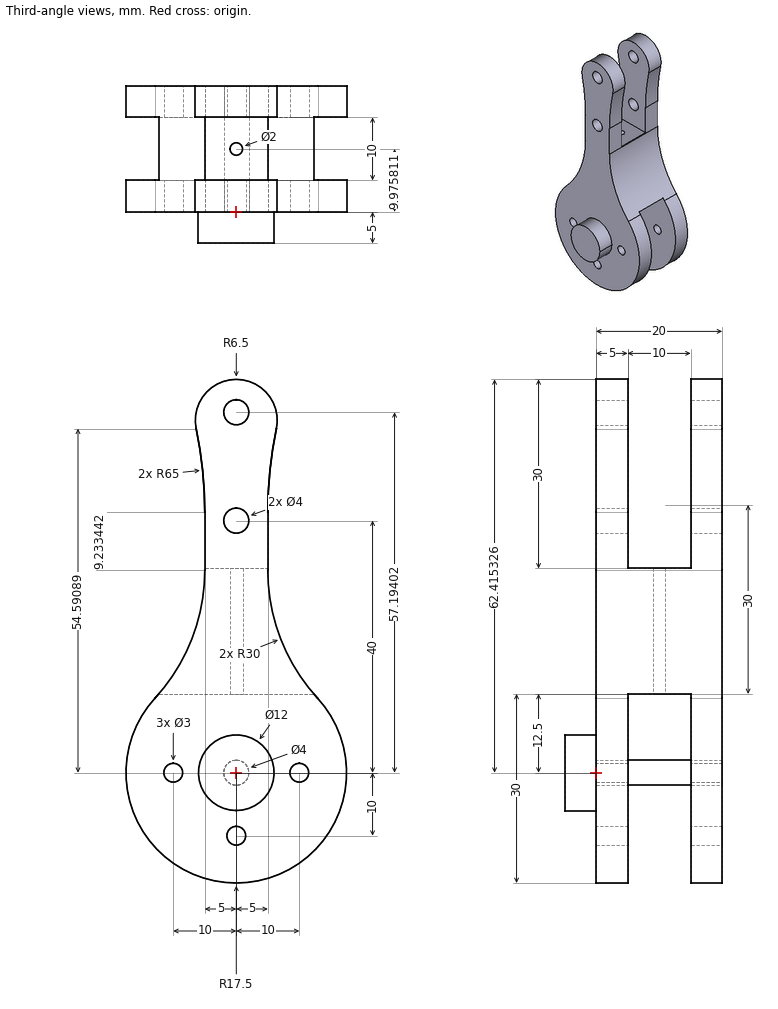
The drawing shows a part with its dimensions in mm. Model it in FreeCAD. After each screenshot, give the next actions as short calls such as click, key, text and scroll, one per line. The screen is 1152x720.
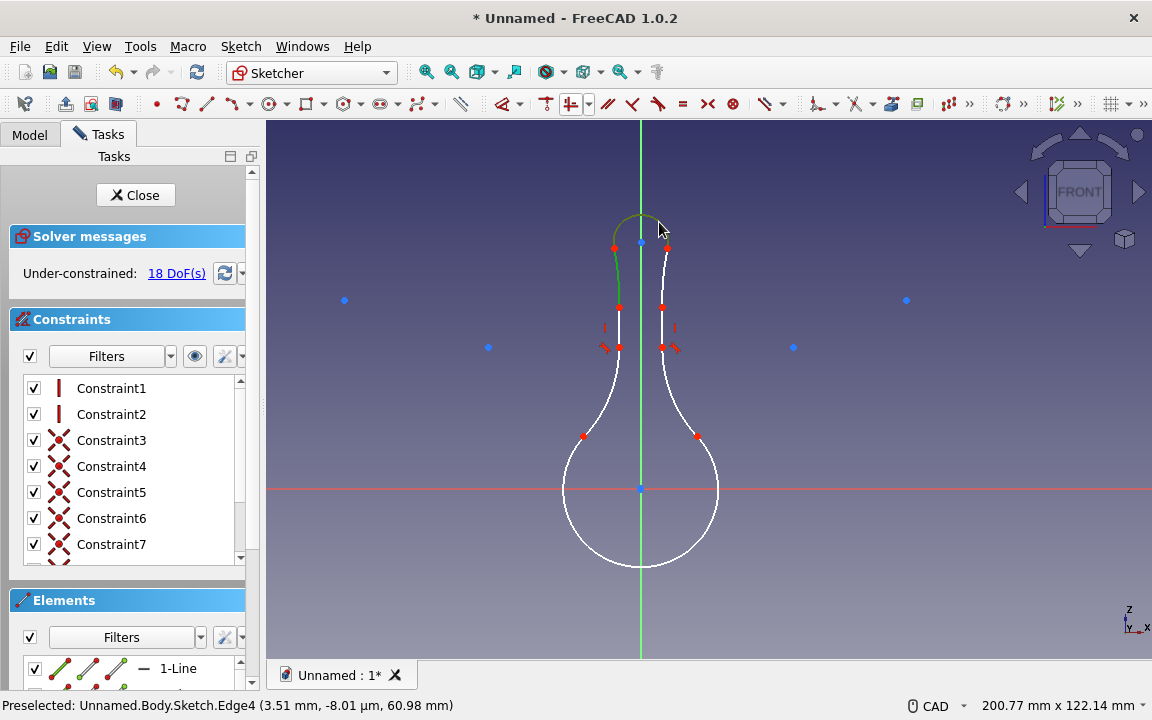
click(658, 104)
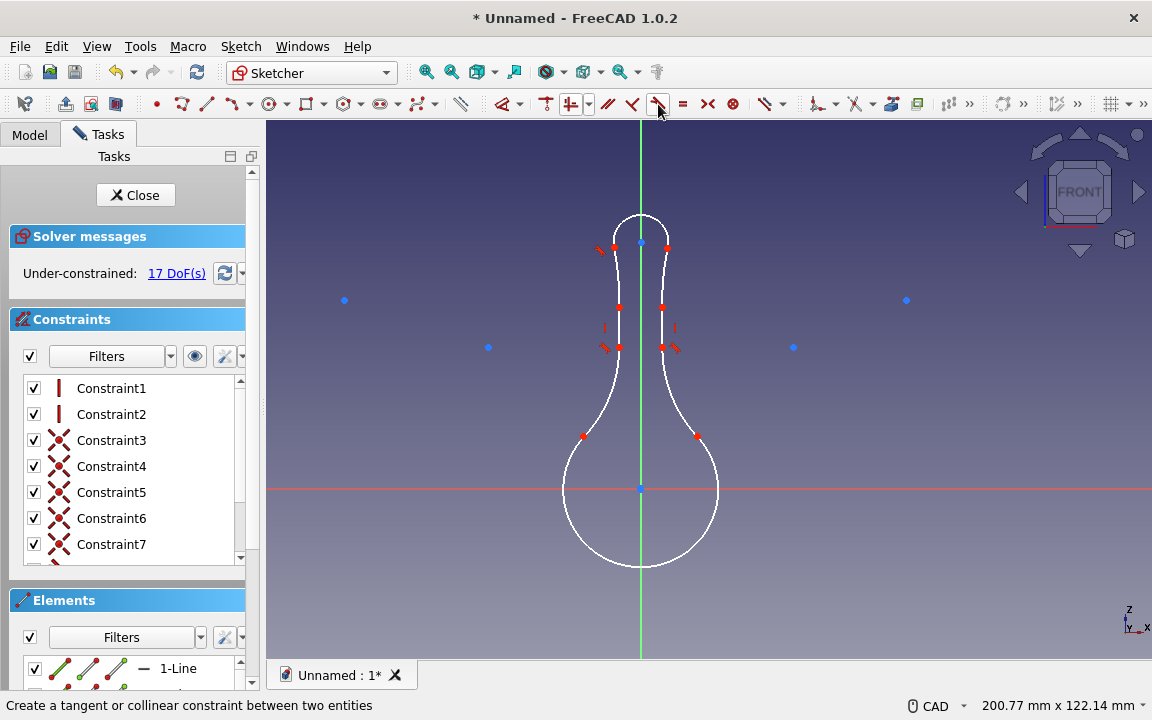
click(660, 222)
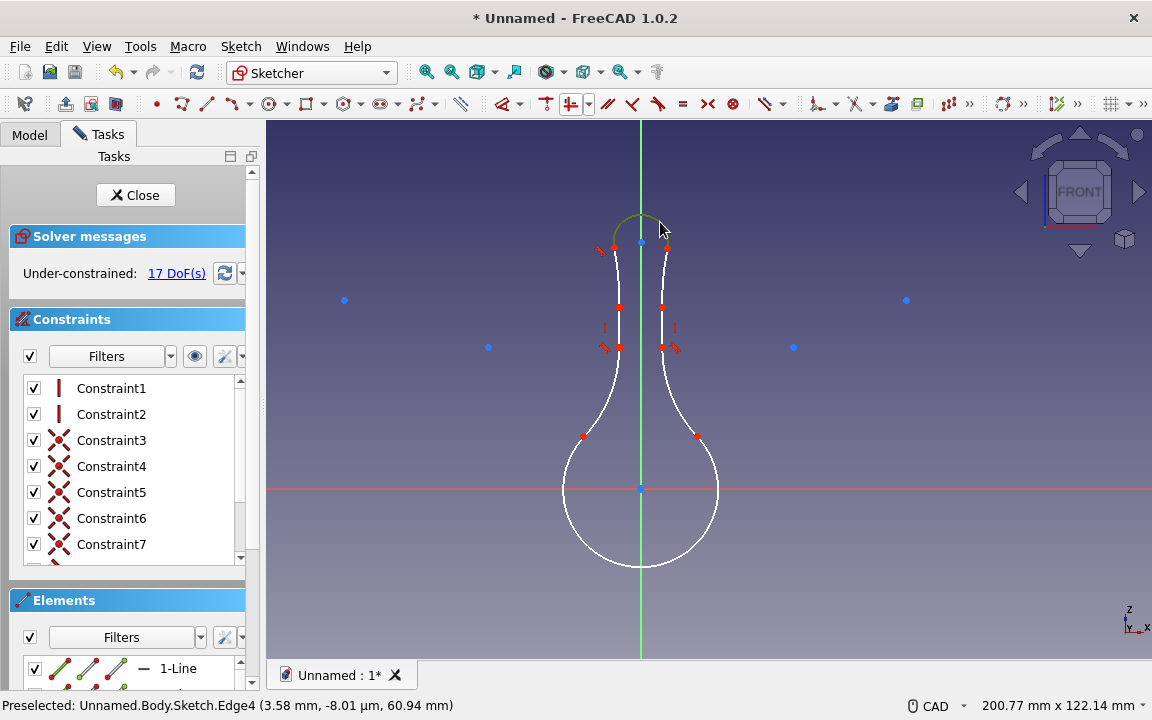
click(665, 266)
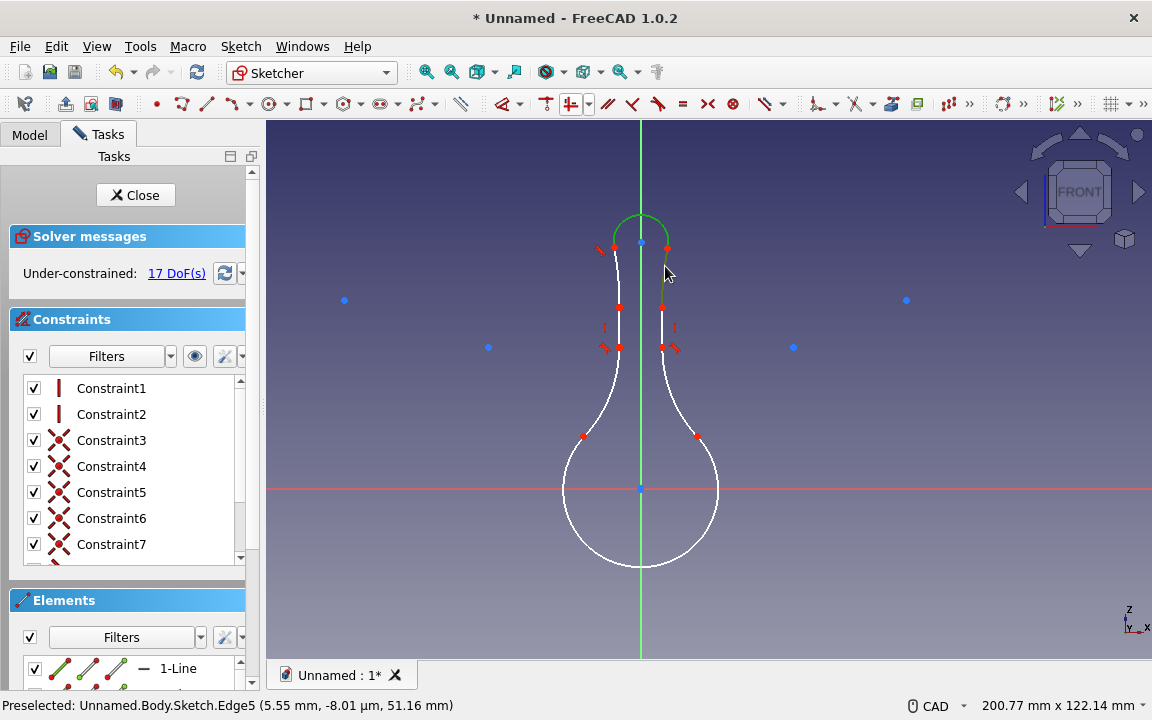
click(658, 104)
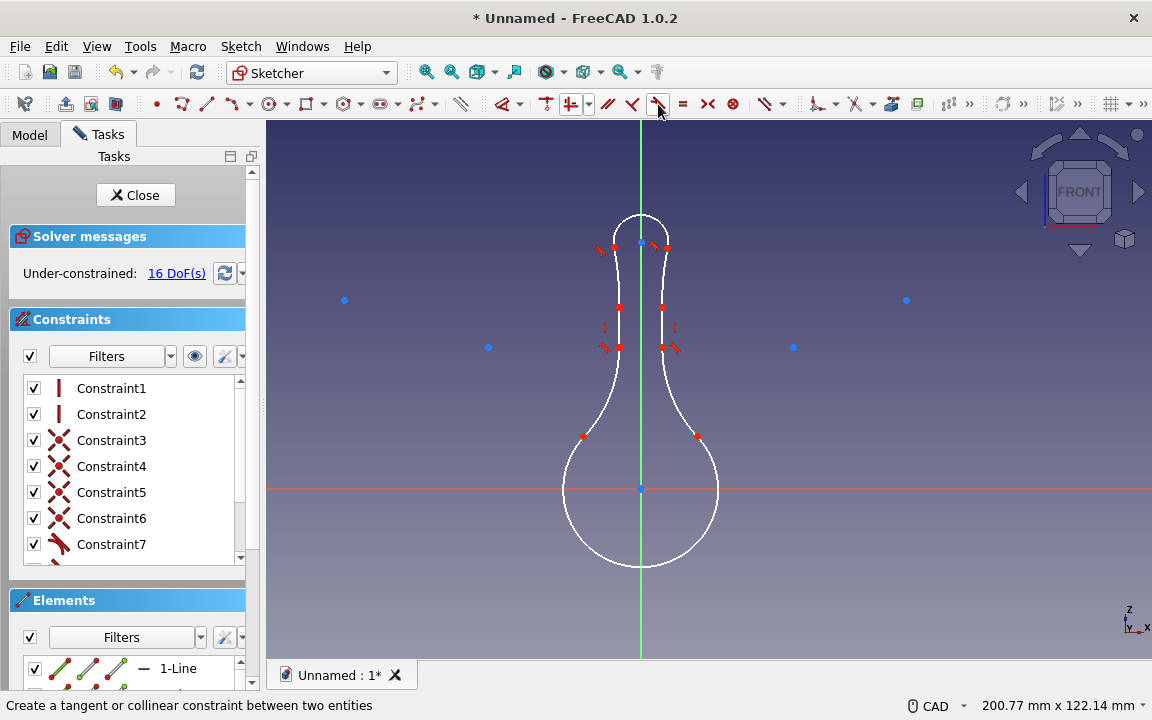
click(666, 377)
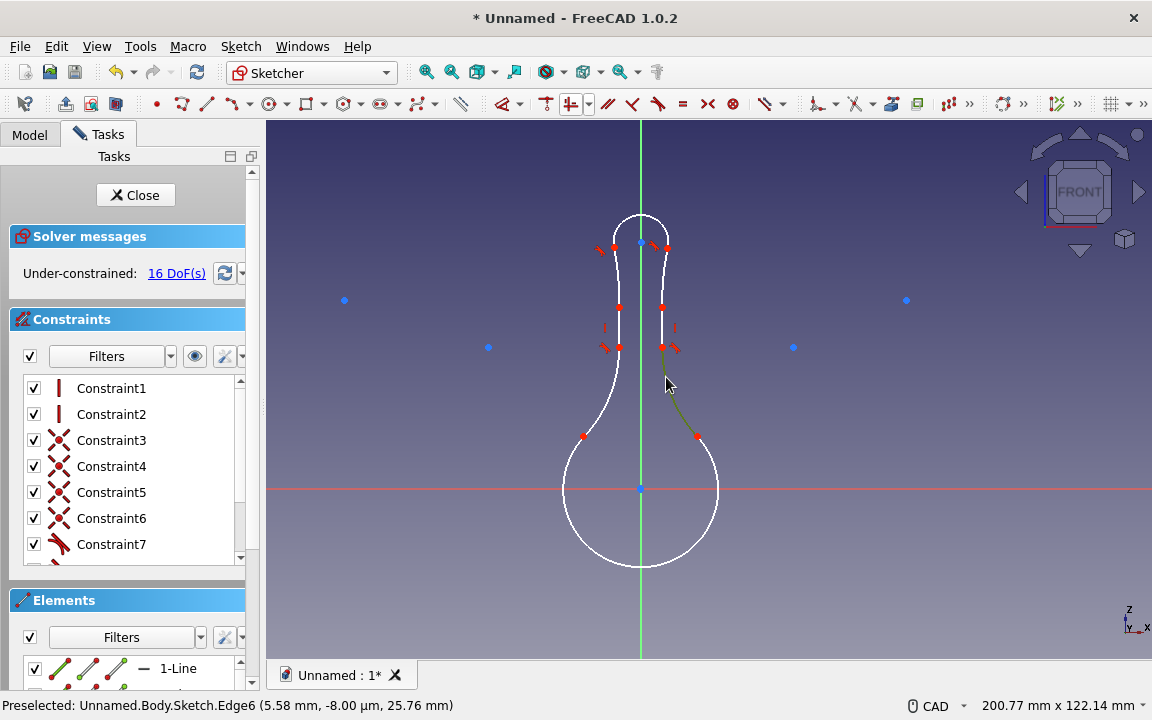
click(579, 536)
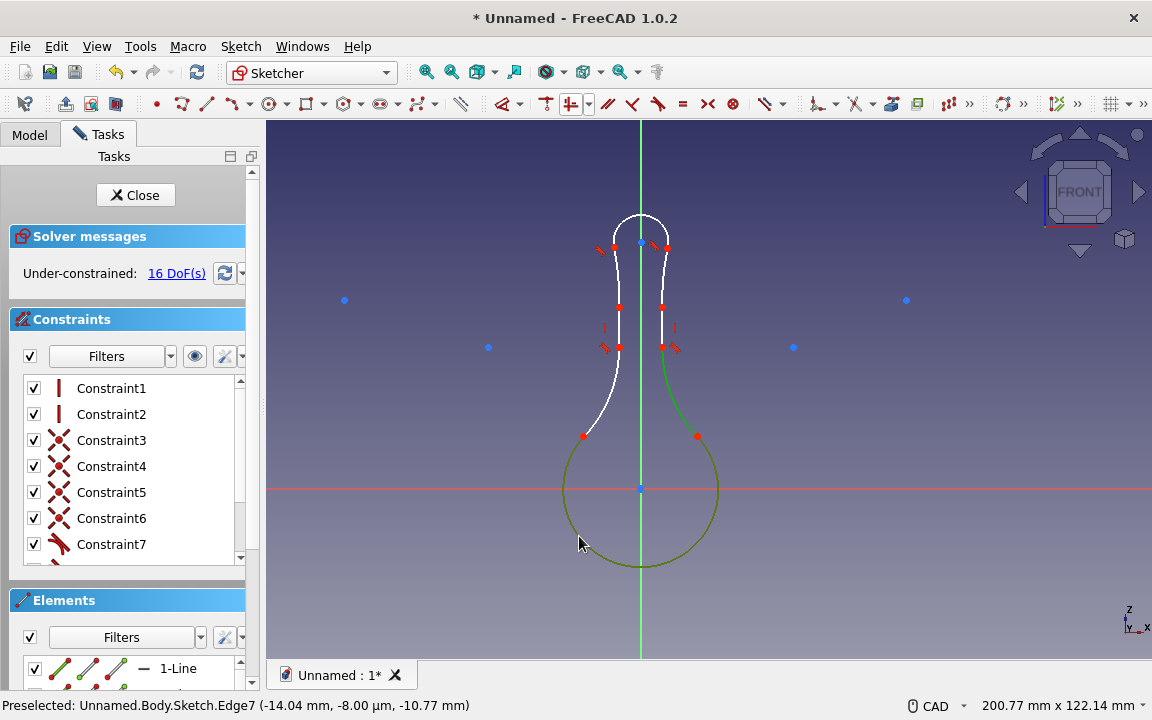
click(658, 104)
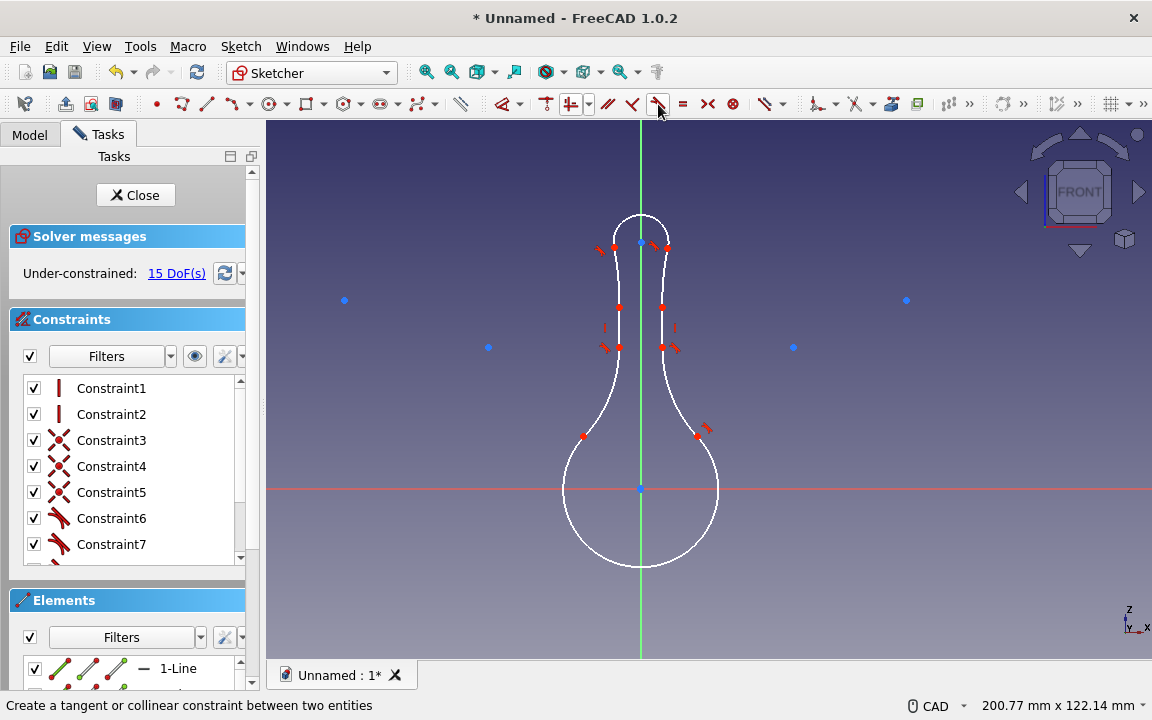
click(579, 536)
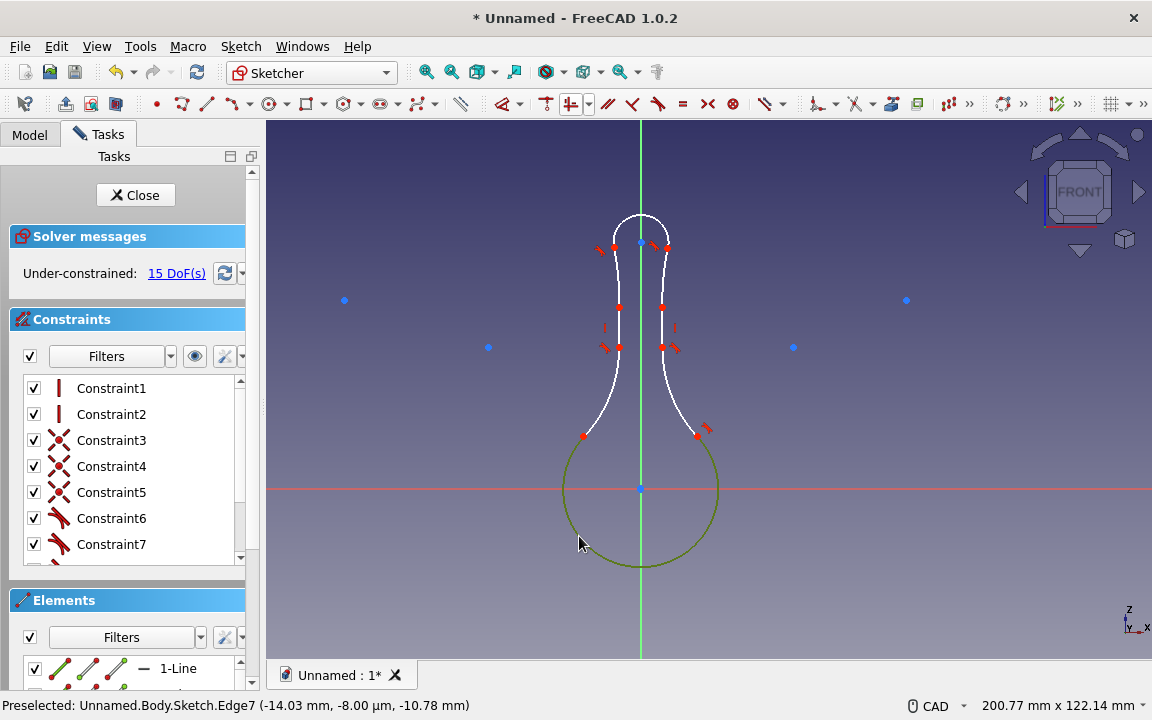
click(601, 413)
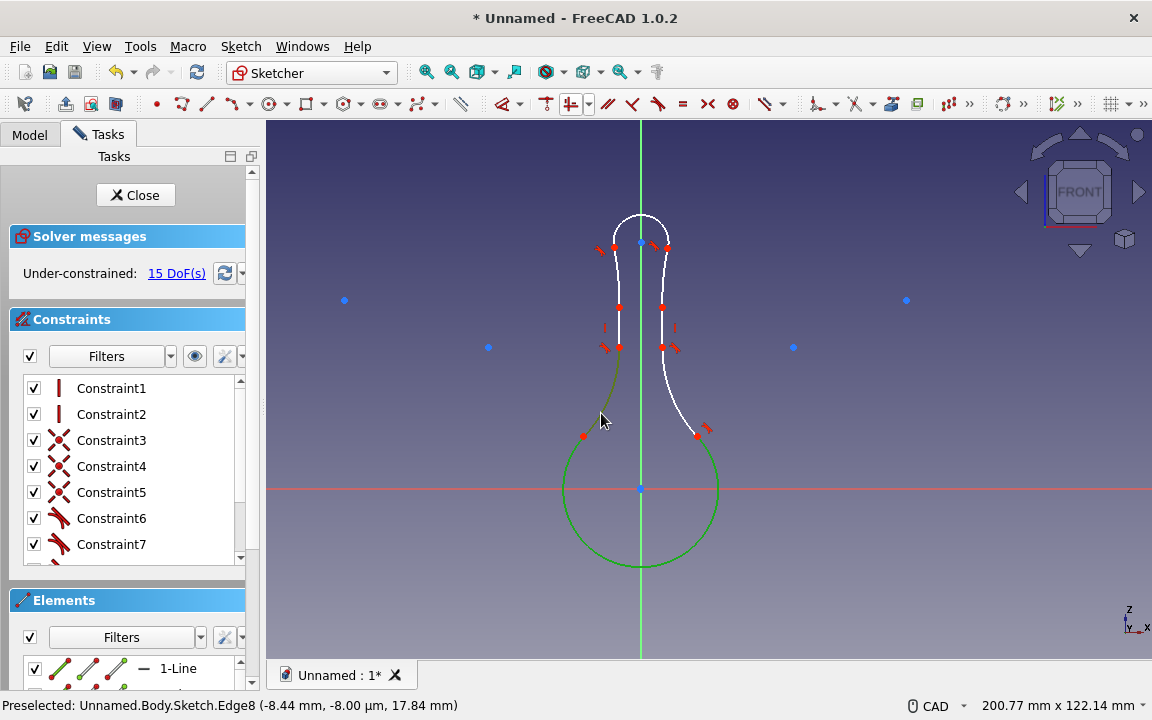
click(658, 104)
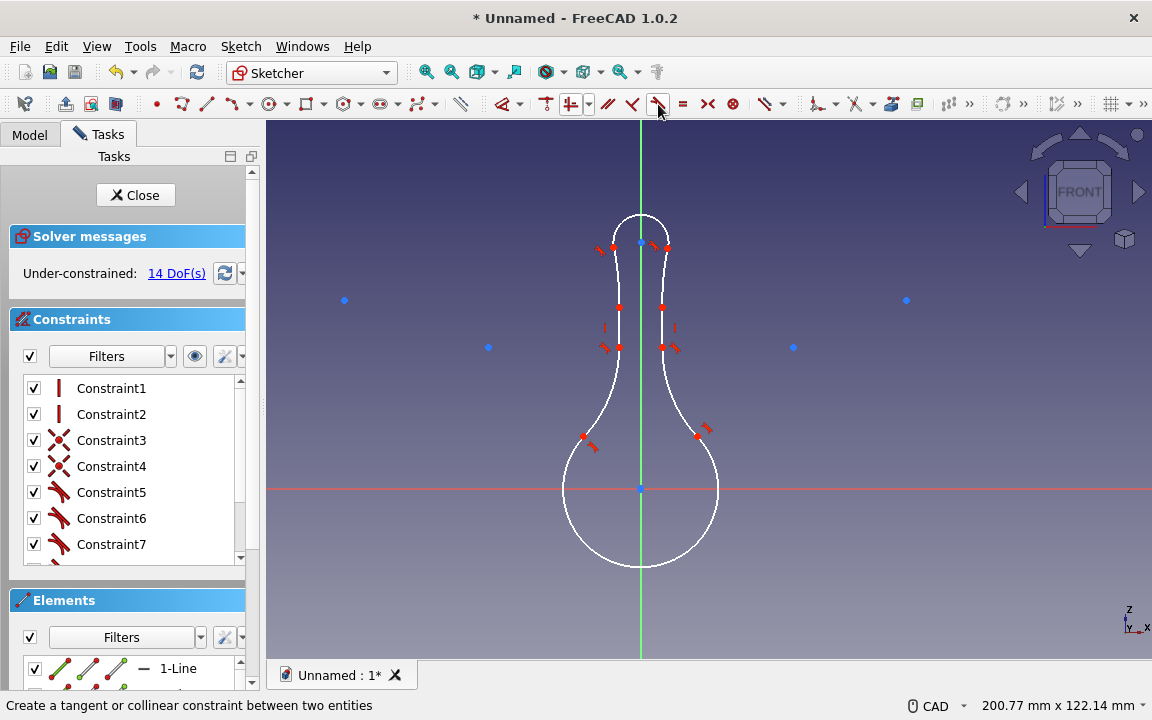
scroll(641, 489, up, 2)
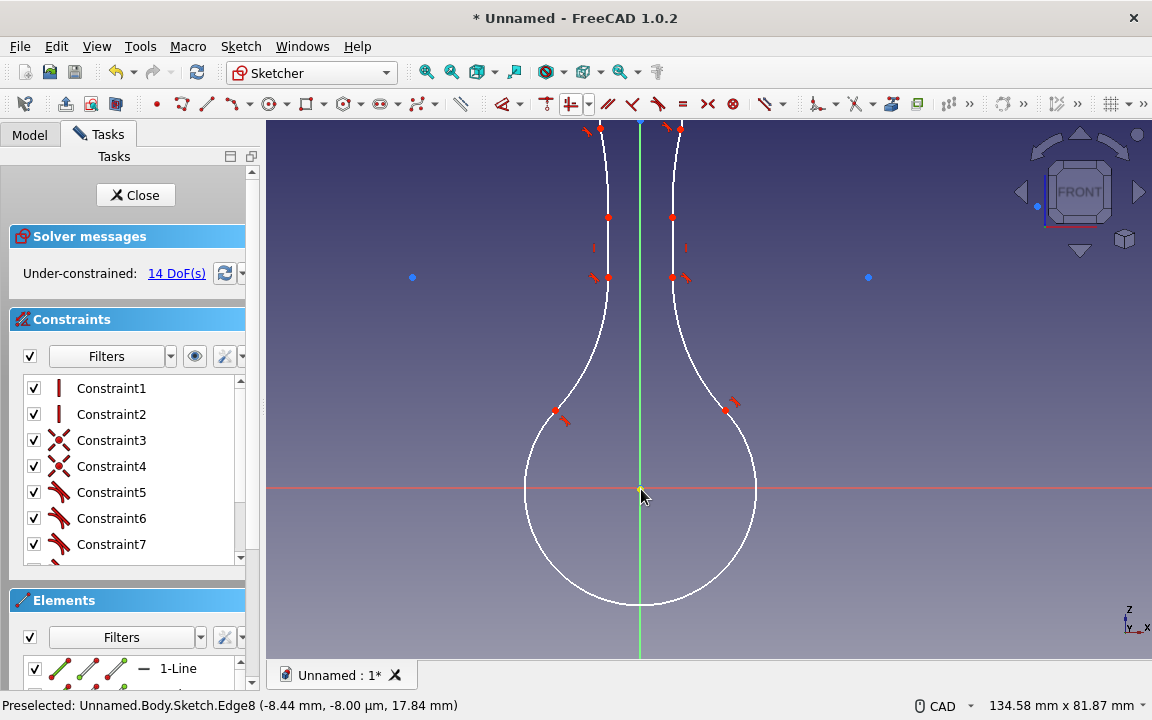
drag(630, 478, 650, 500)